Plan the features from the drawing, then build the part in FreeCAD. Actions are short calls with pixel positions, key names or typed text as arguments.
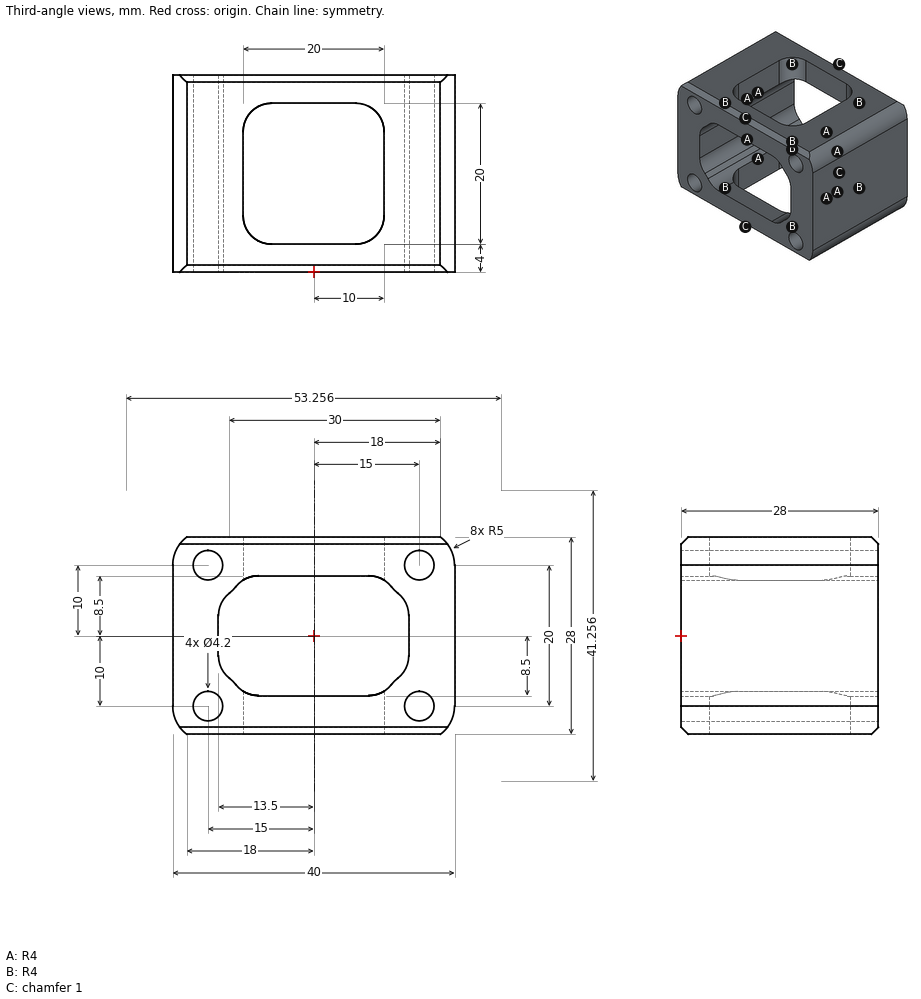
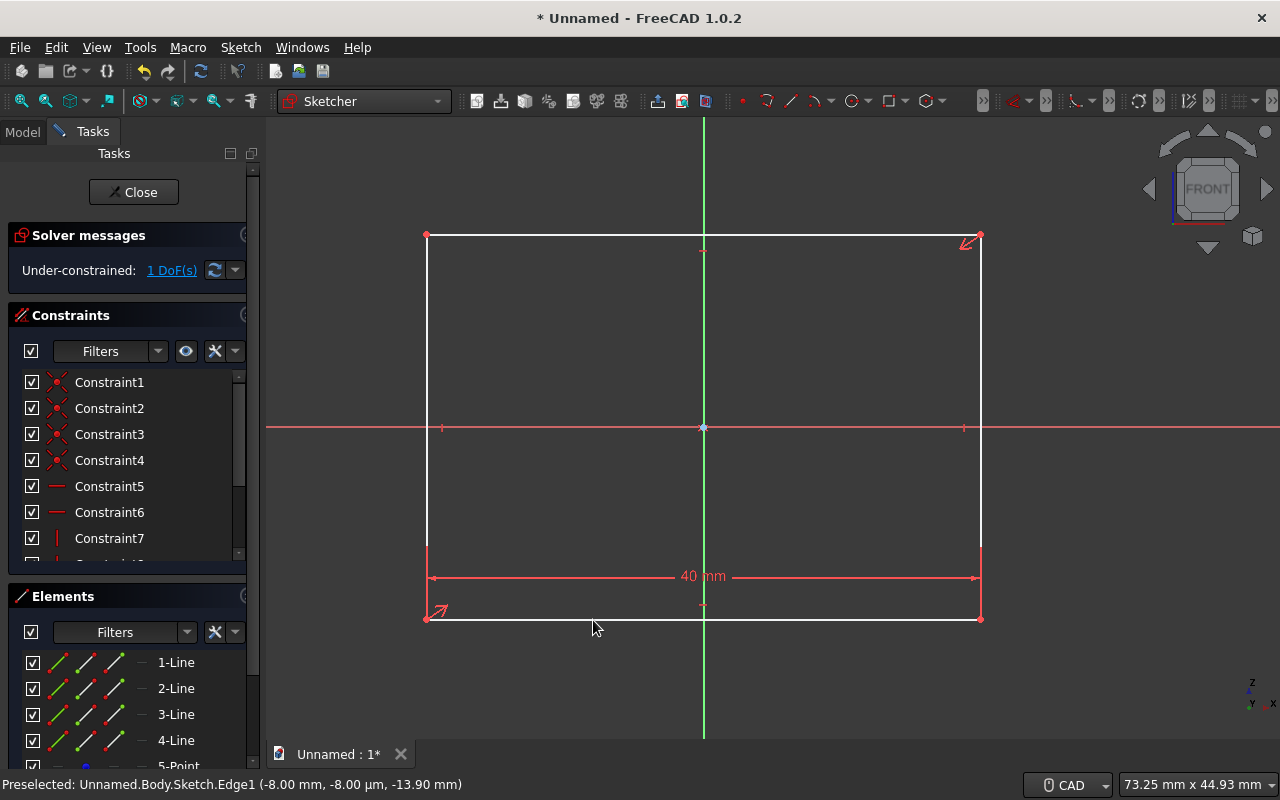
click(981, 504)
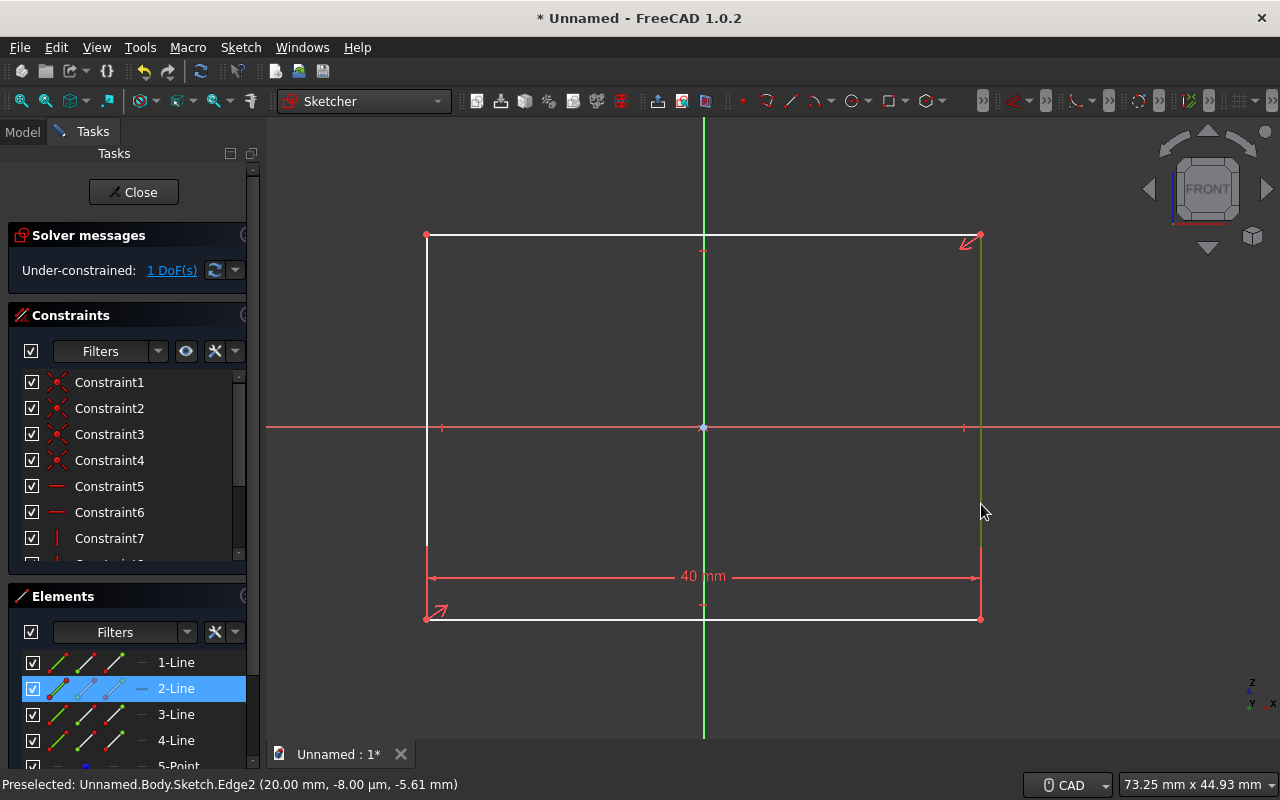
key(i)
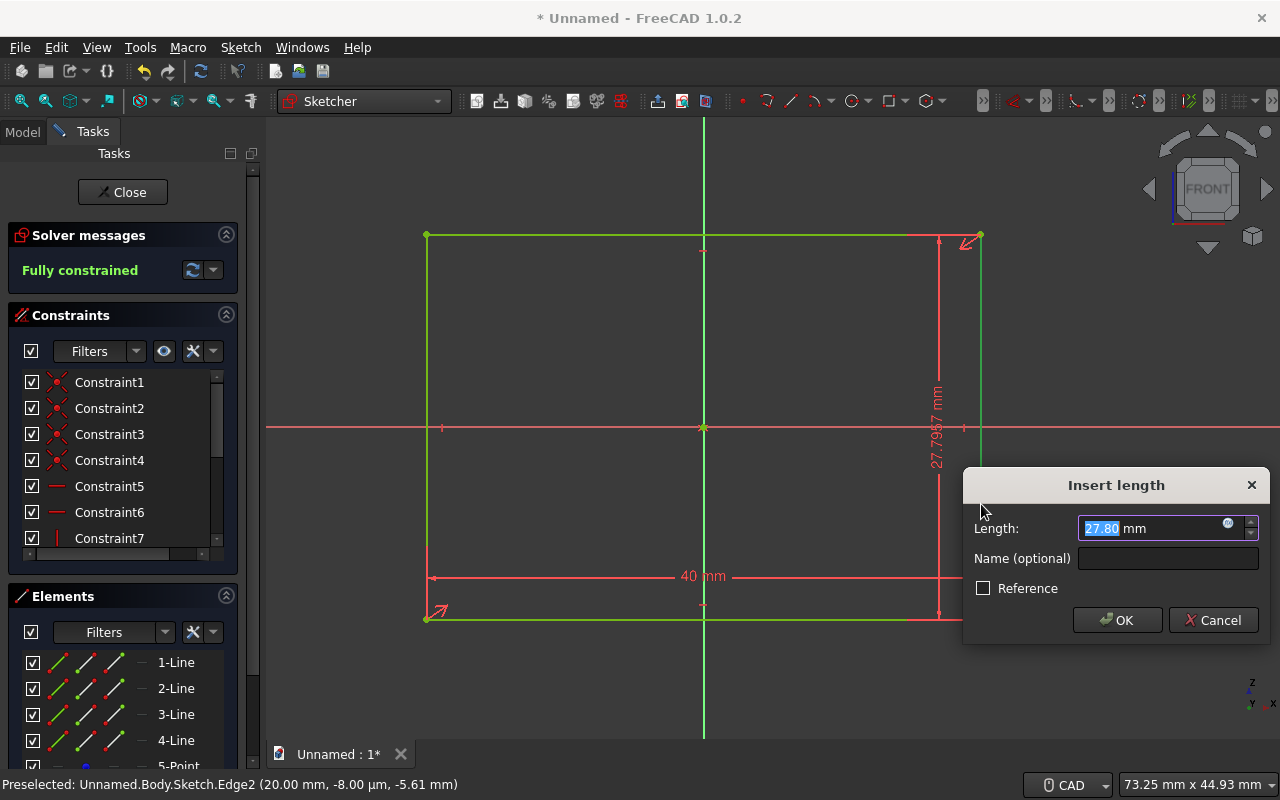
text(28)
key(Return)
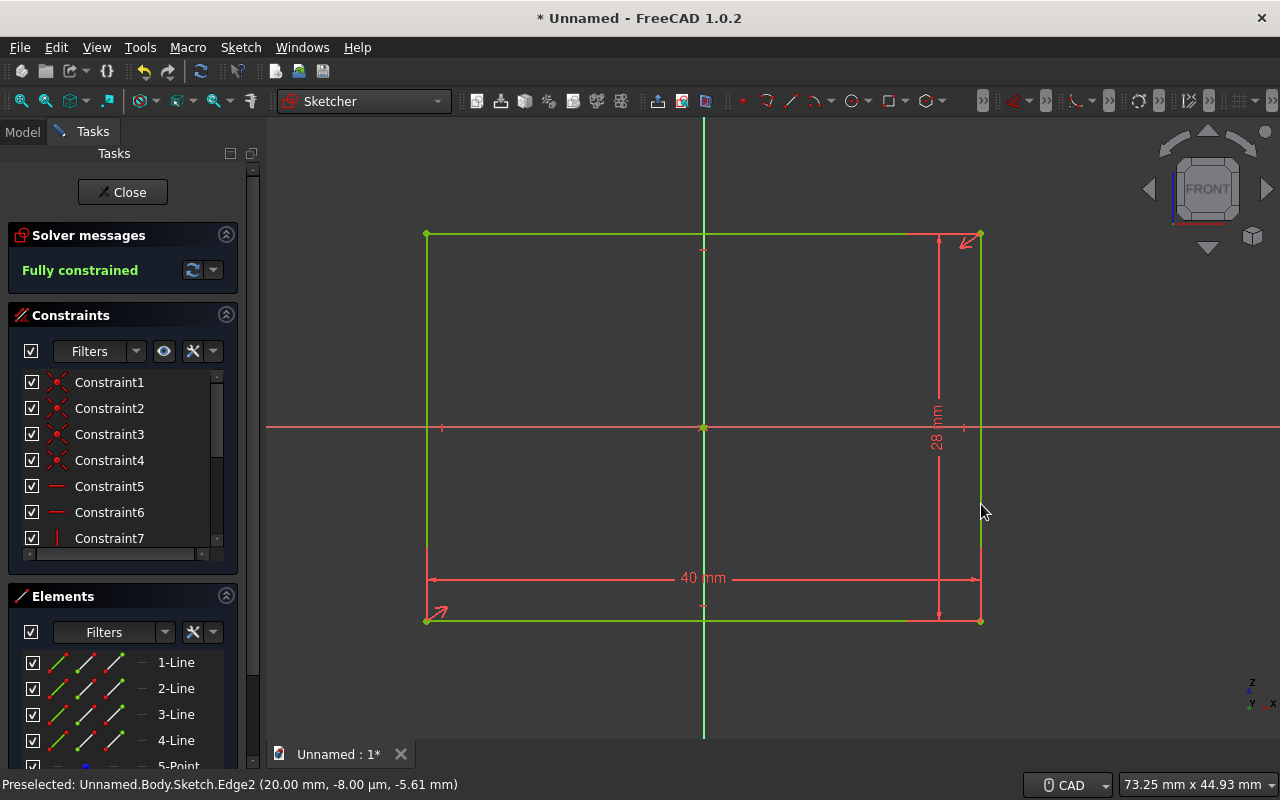
click(123, 192)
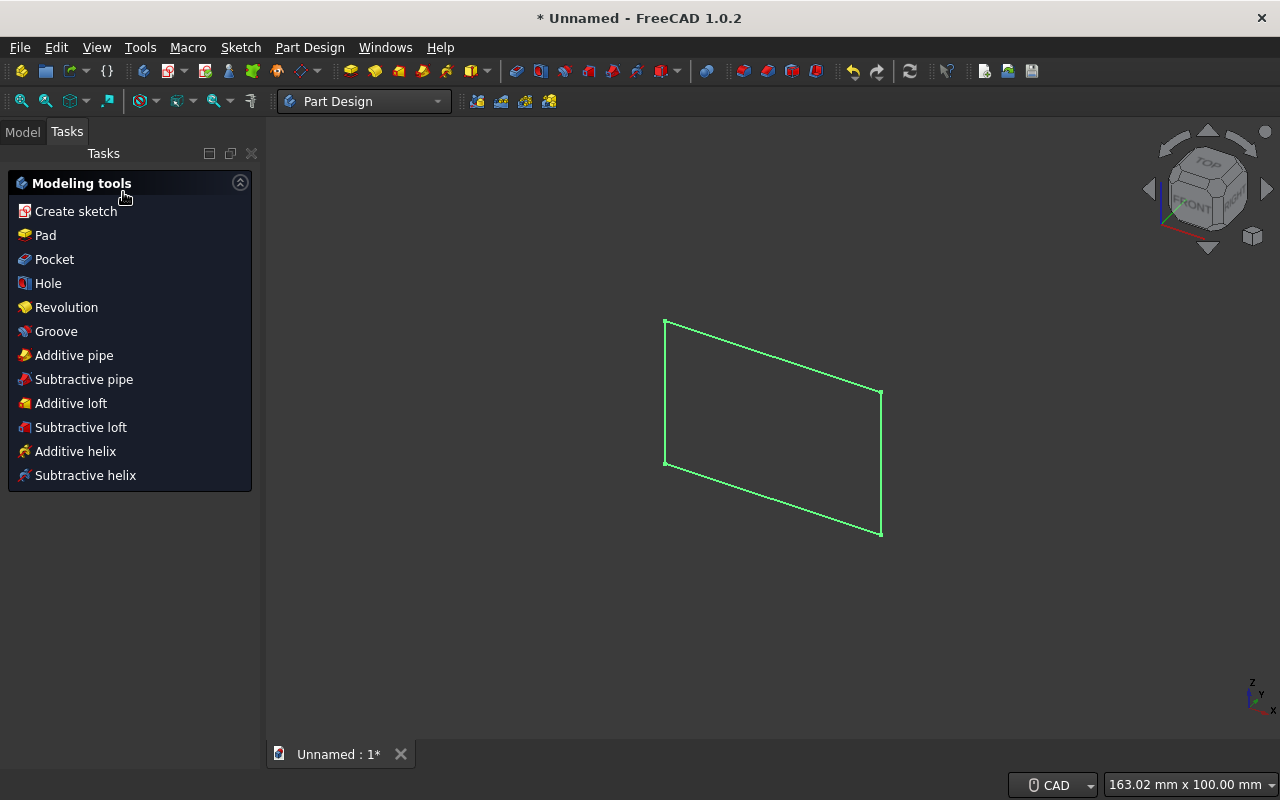
click(352, 72)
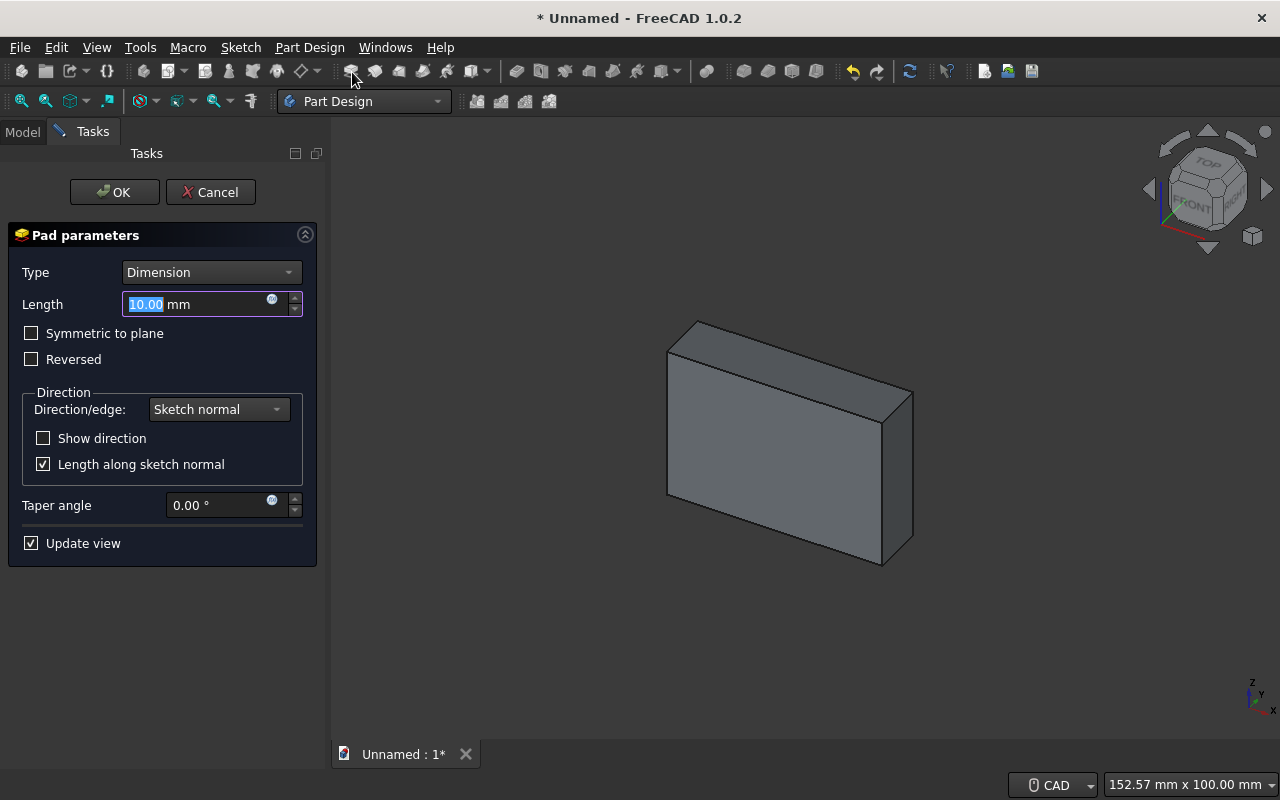
text(28)
key(Tab)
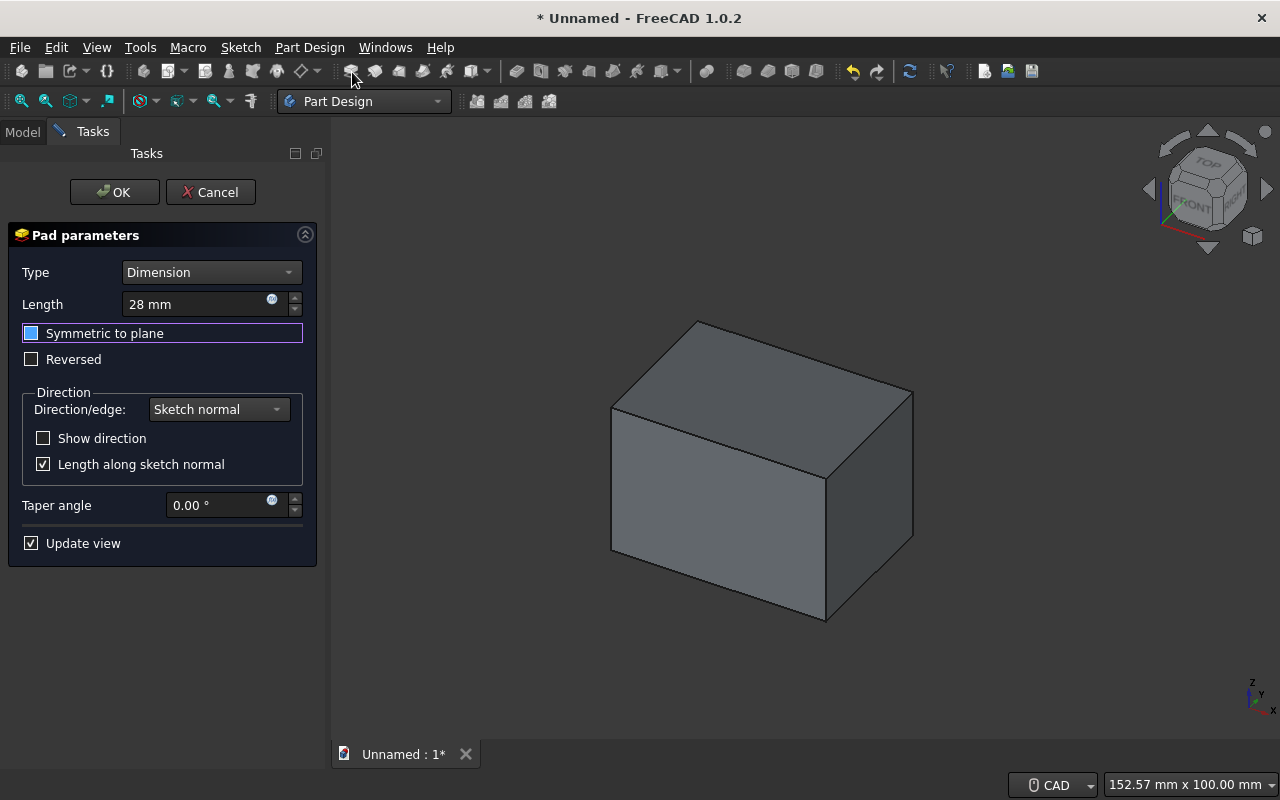
click(30, 359)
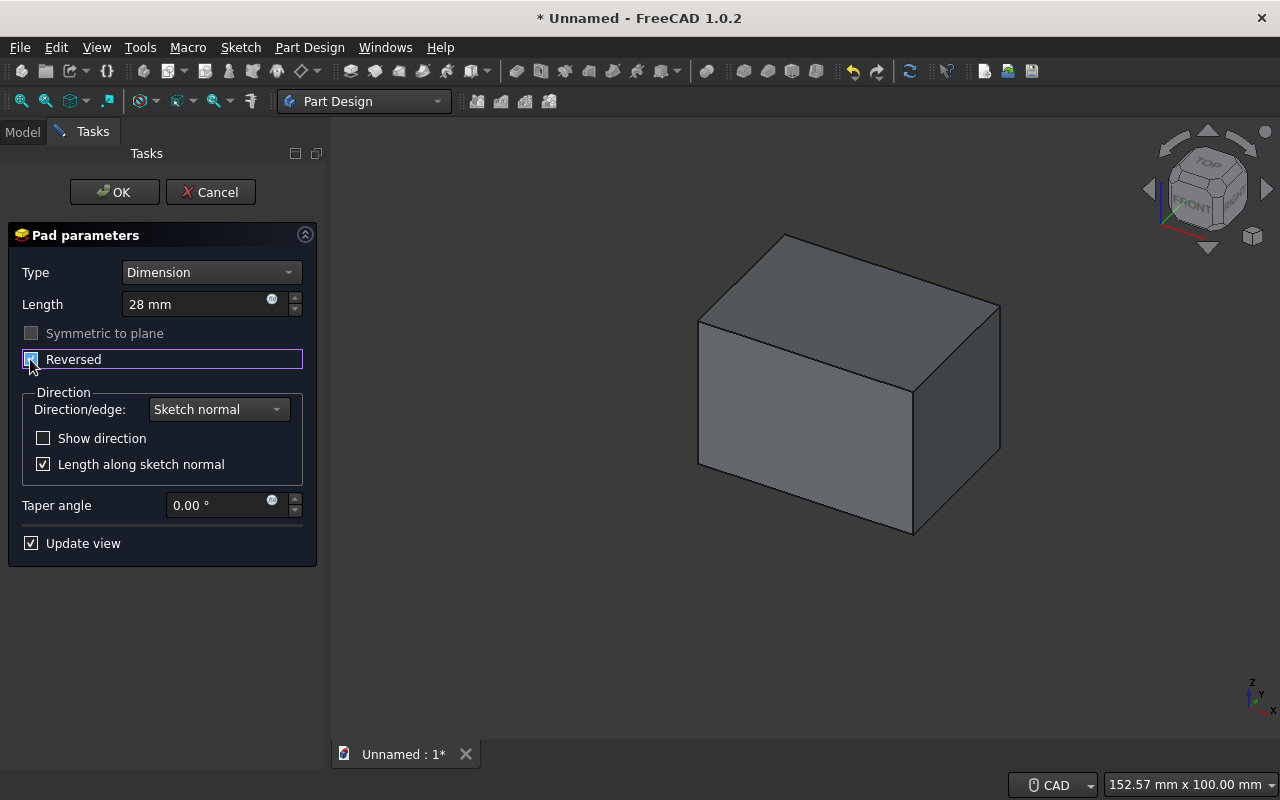
click(115, 192)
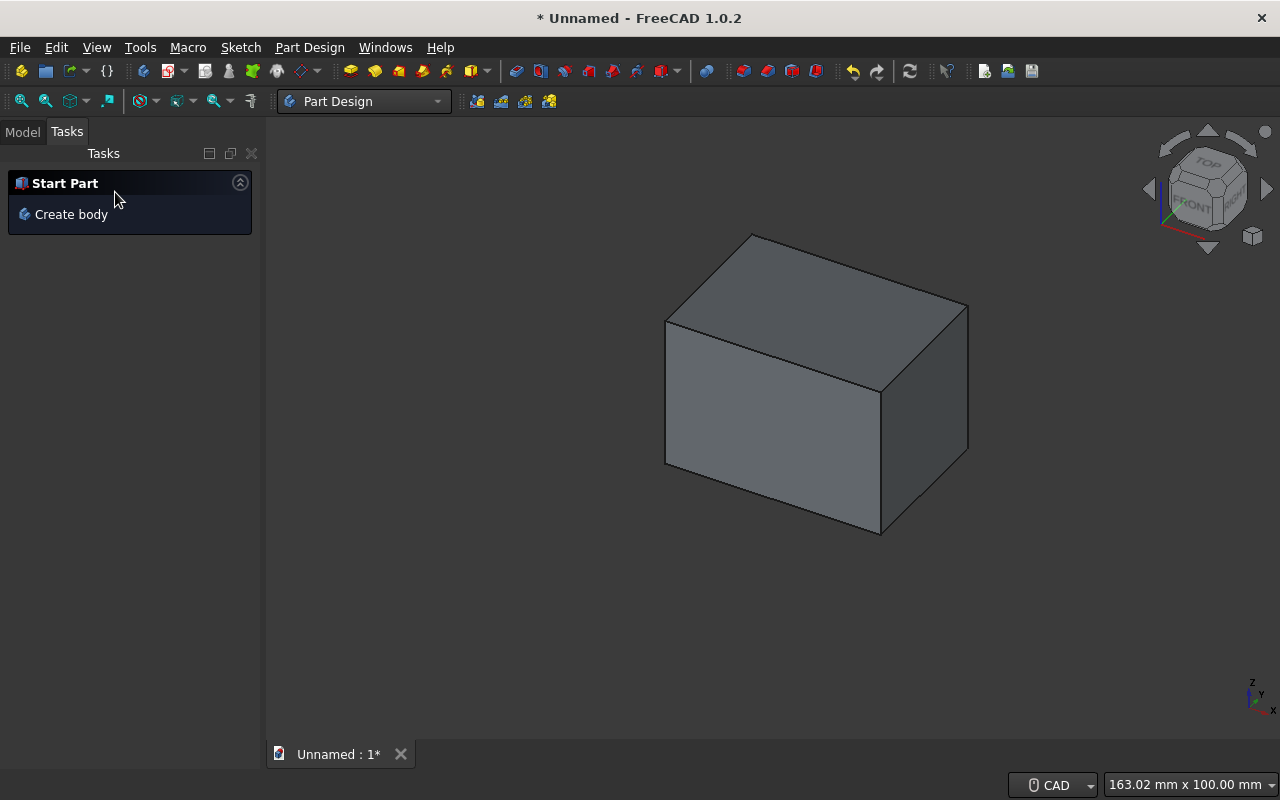
key(4)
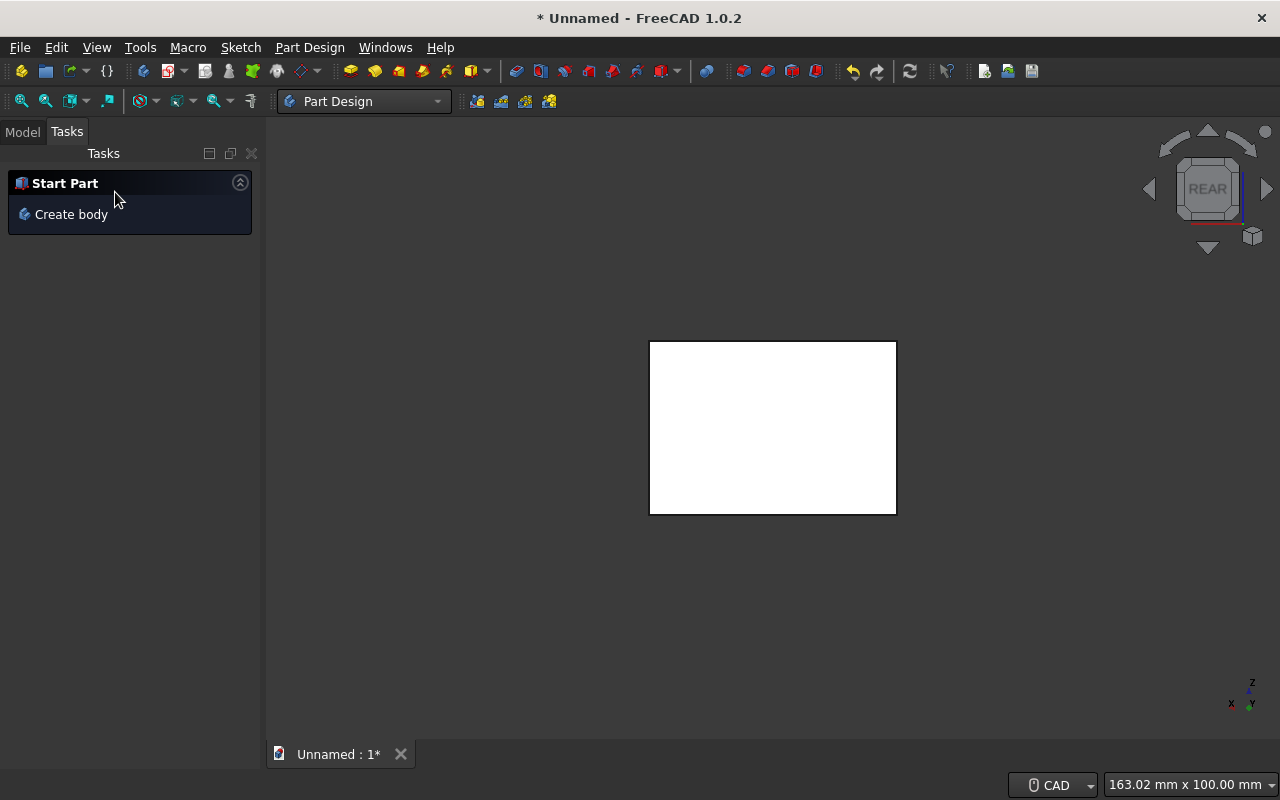
key(v)
key(f)